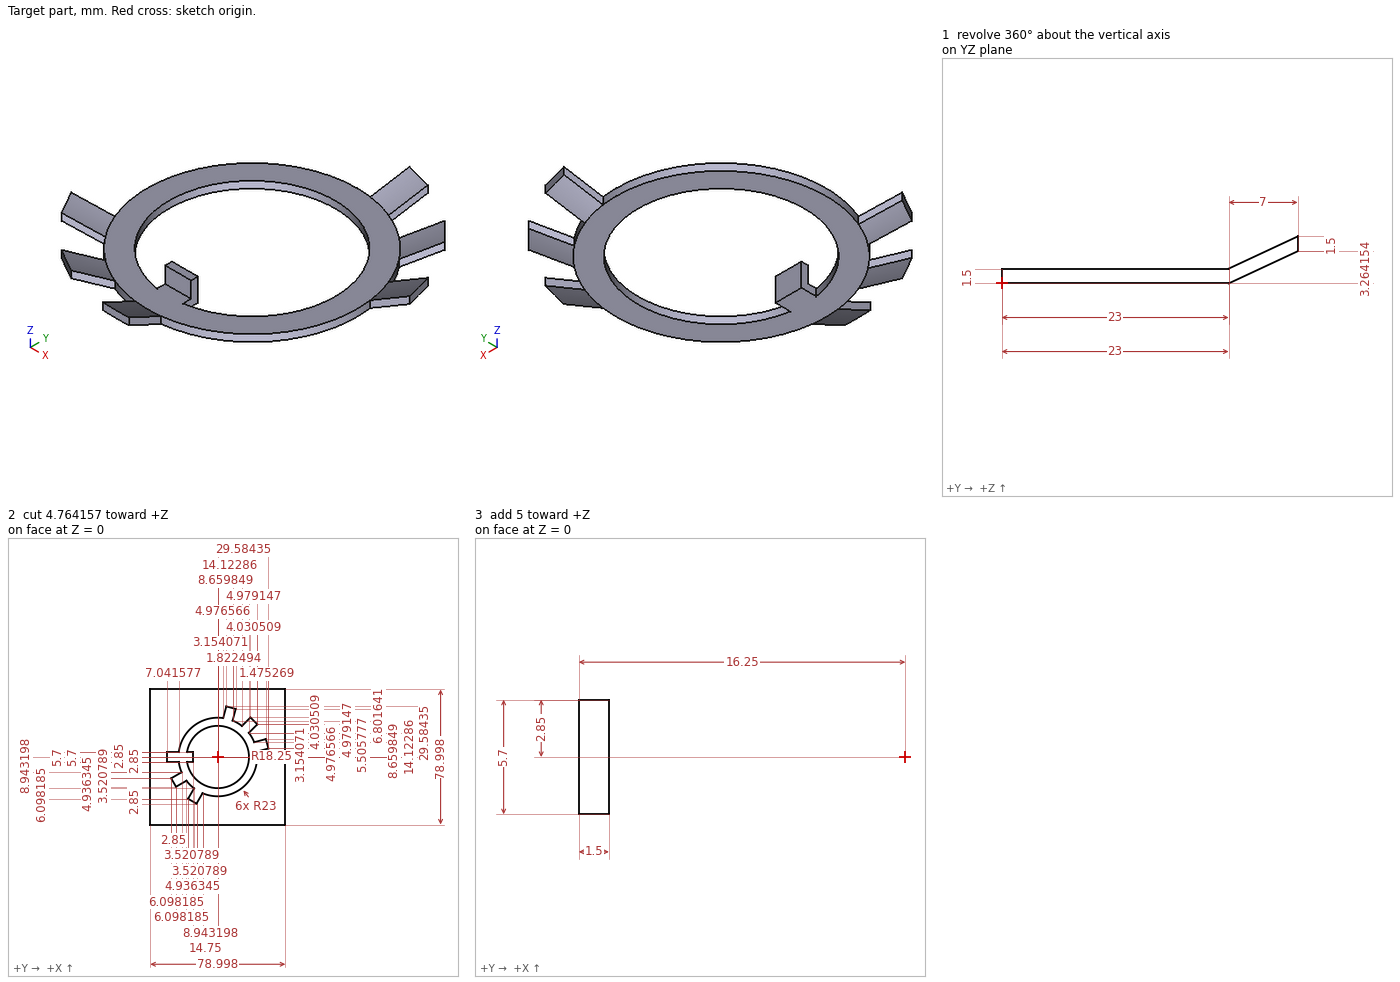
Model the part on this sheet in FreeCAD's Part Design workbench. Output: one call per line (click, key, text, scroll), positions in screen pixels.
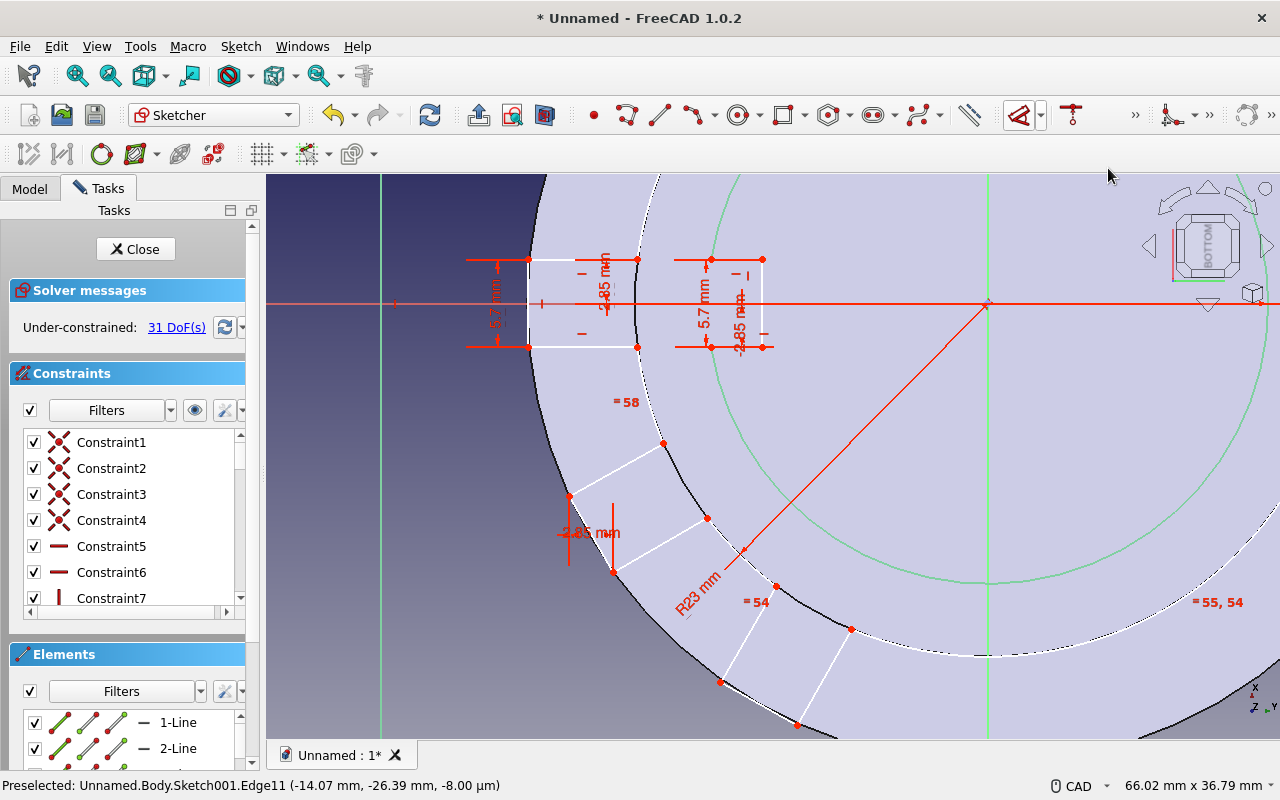
click(744, 695)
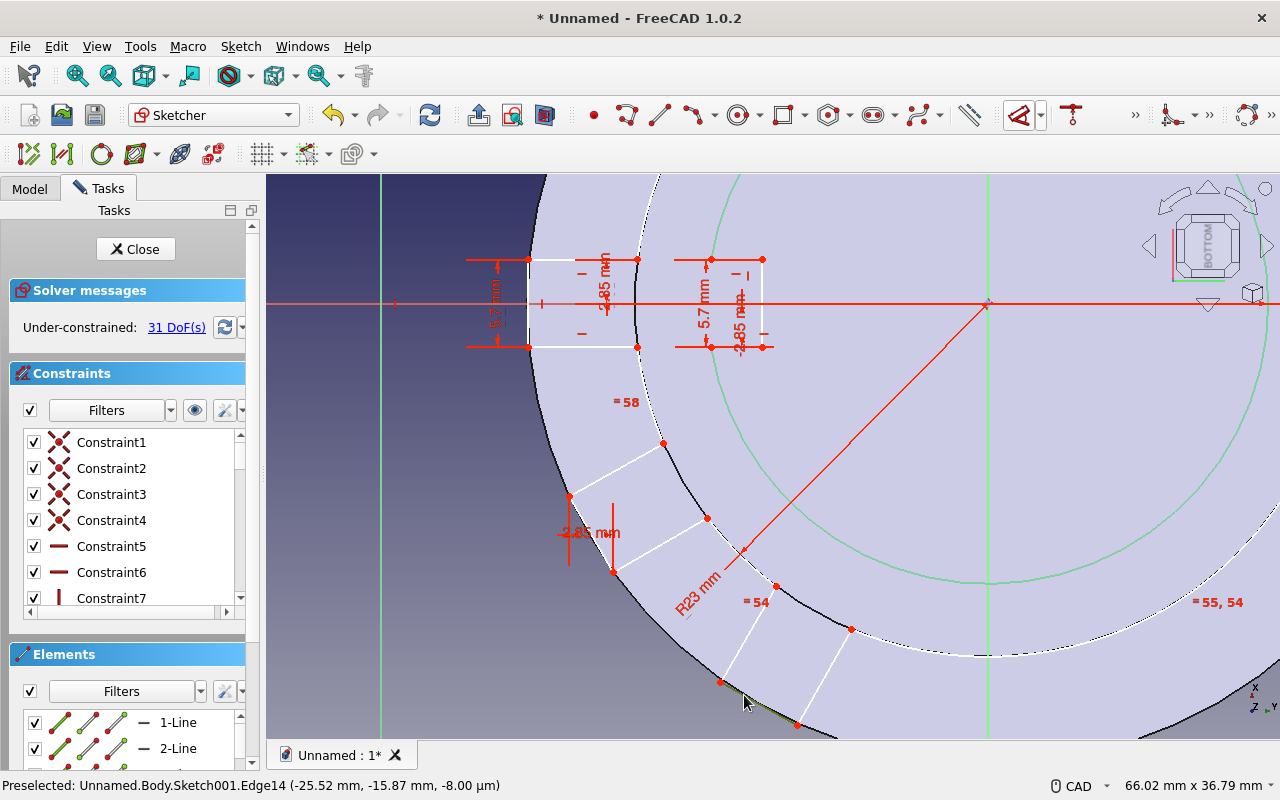
click(1040, 116)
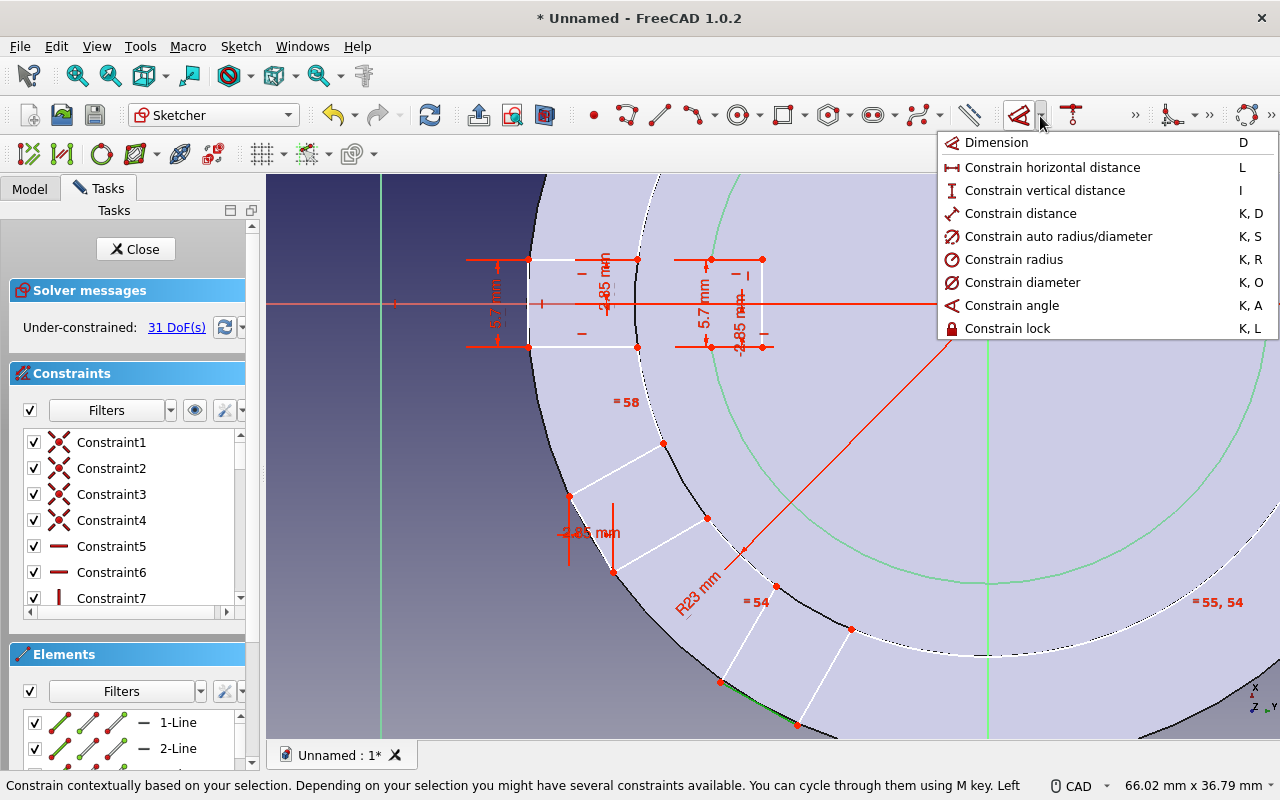
click(1108, 190)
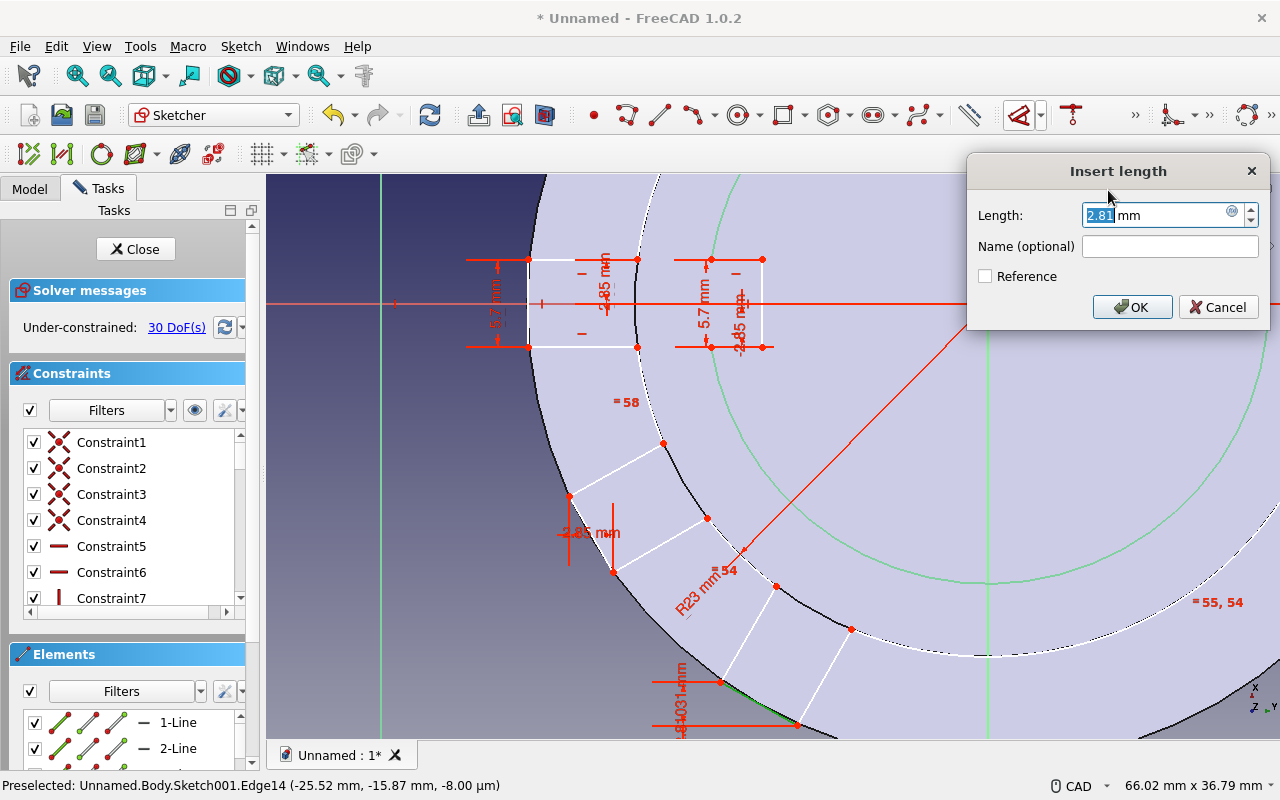
text(2.85)
key(Return)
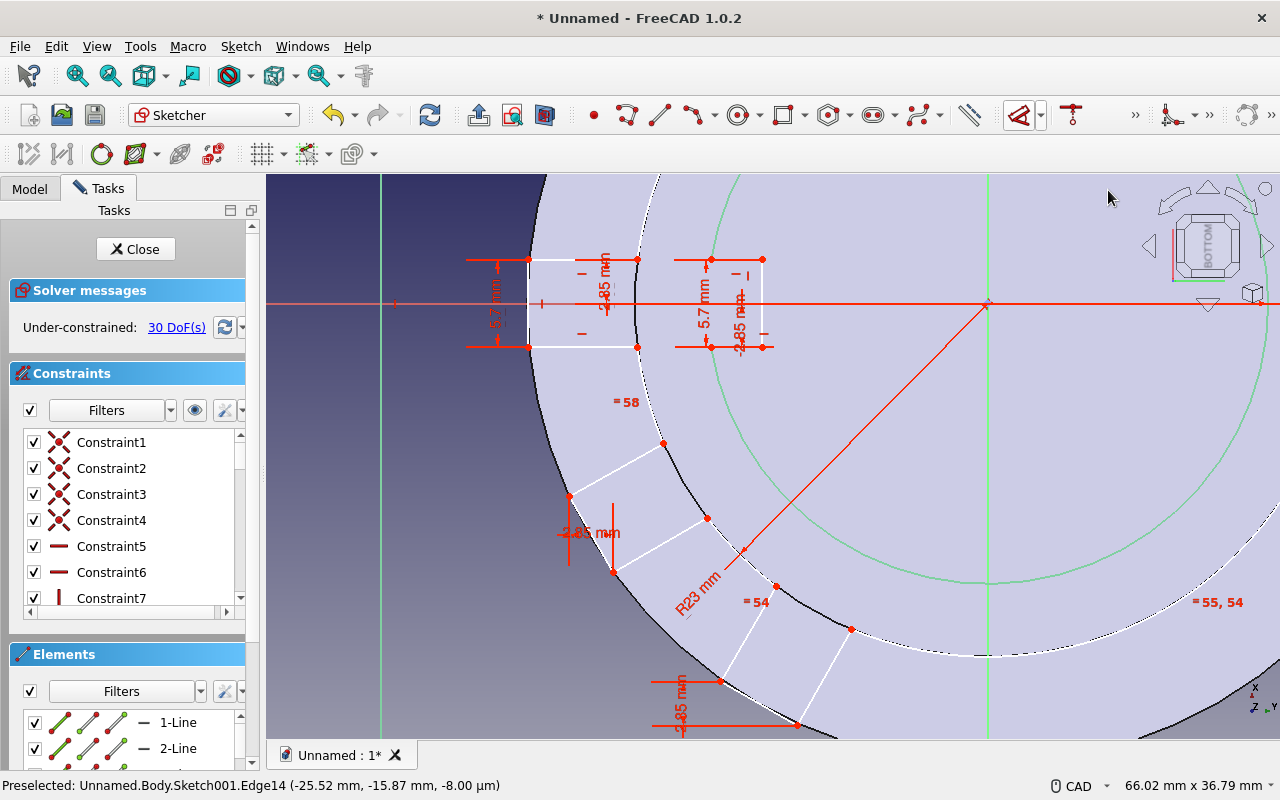
click(762, 347)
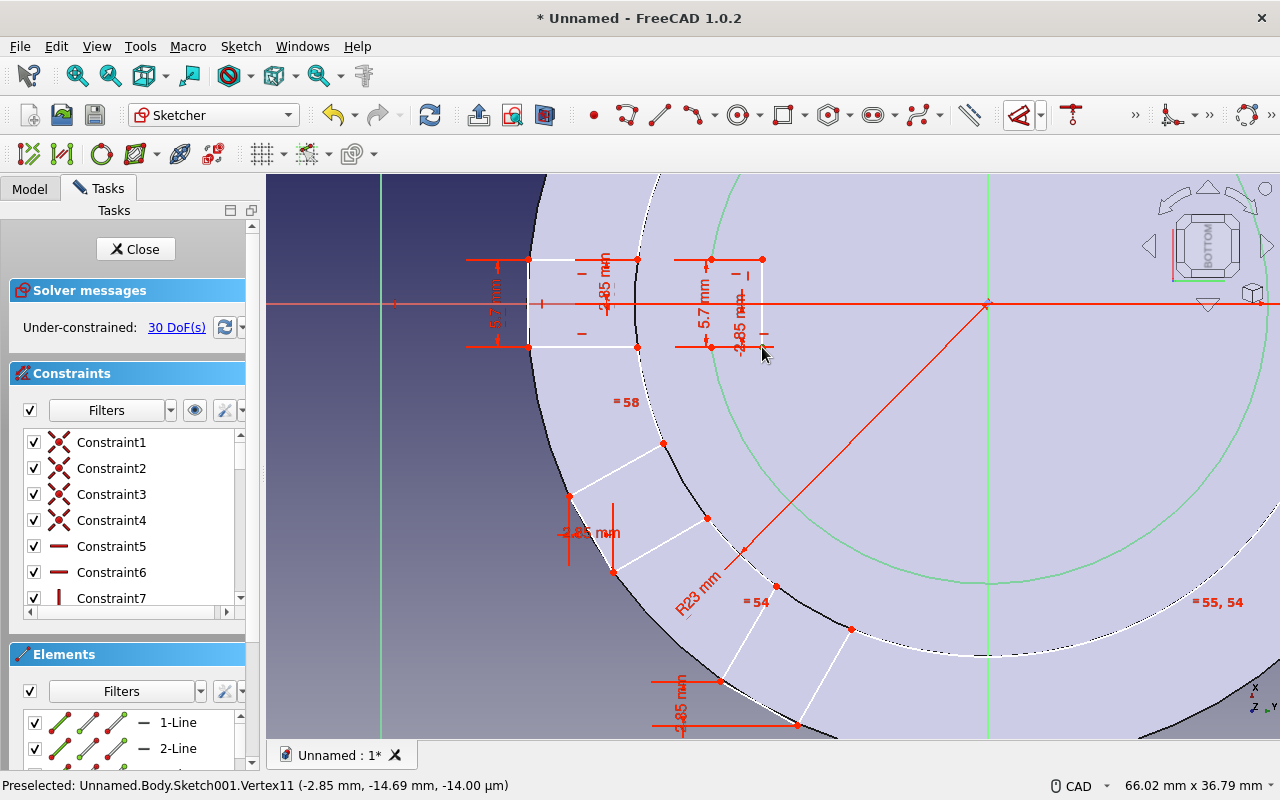
key(l)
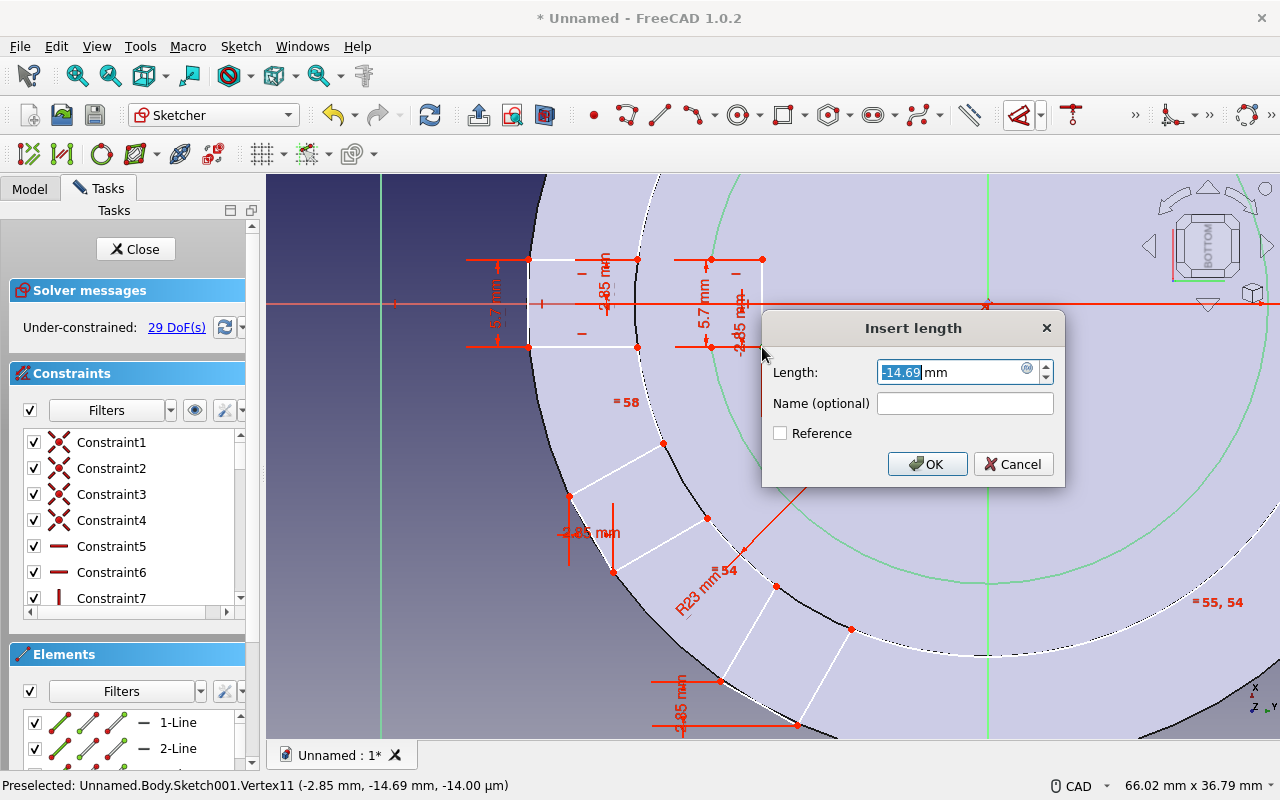
text(-14.75)
key(Return)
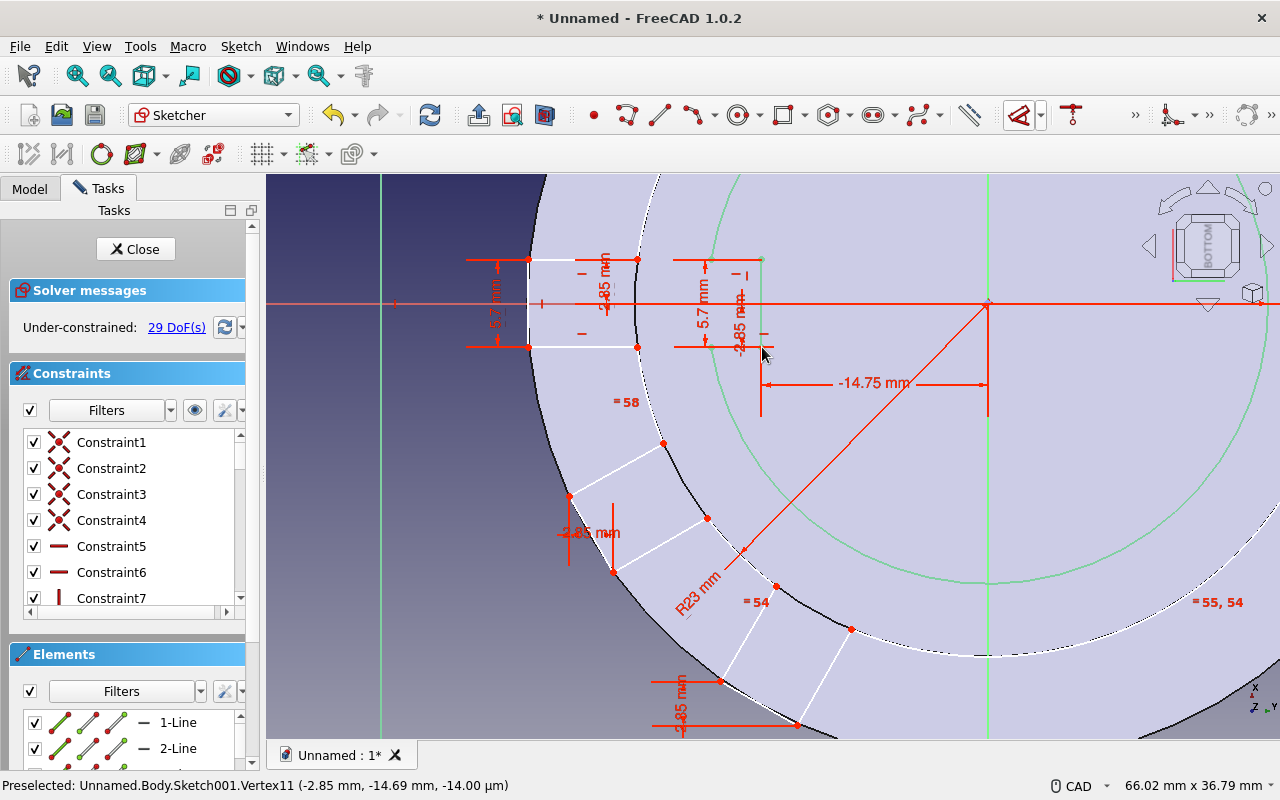
click(561, 260)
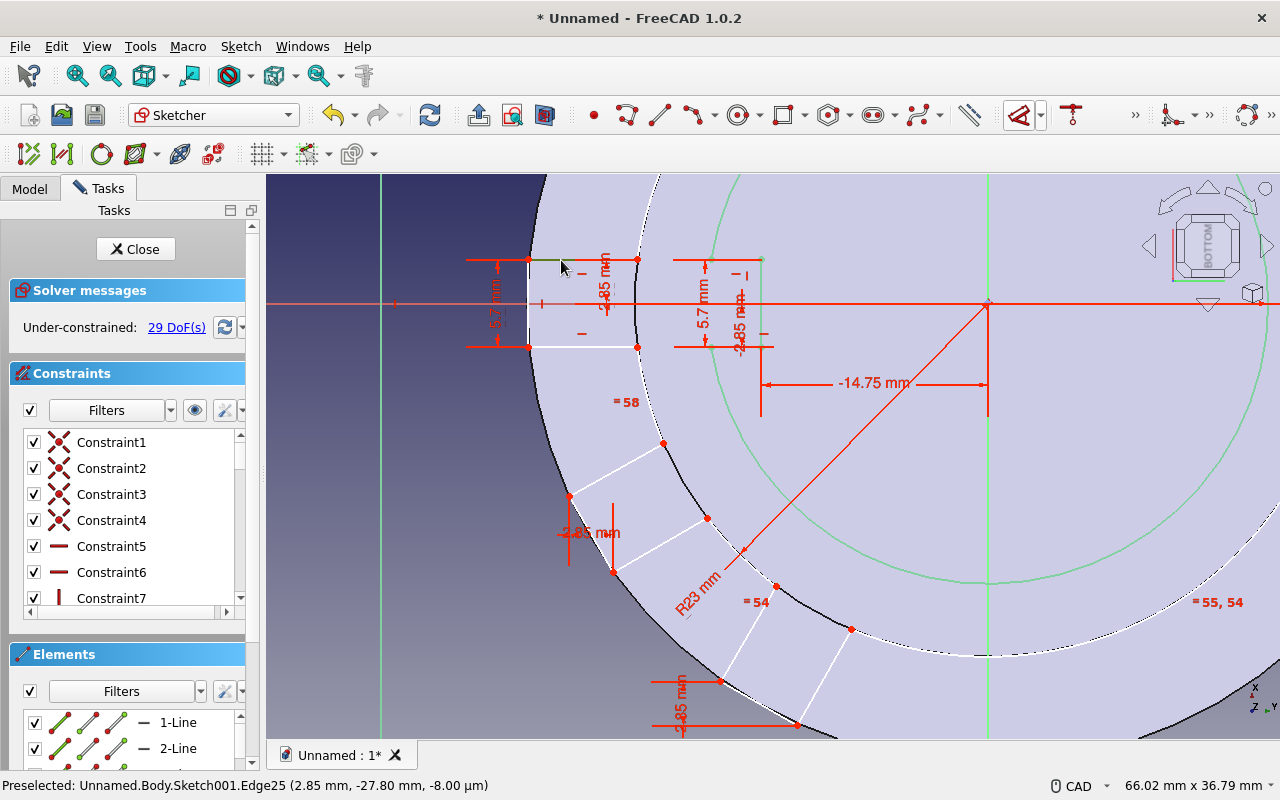
key(l)